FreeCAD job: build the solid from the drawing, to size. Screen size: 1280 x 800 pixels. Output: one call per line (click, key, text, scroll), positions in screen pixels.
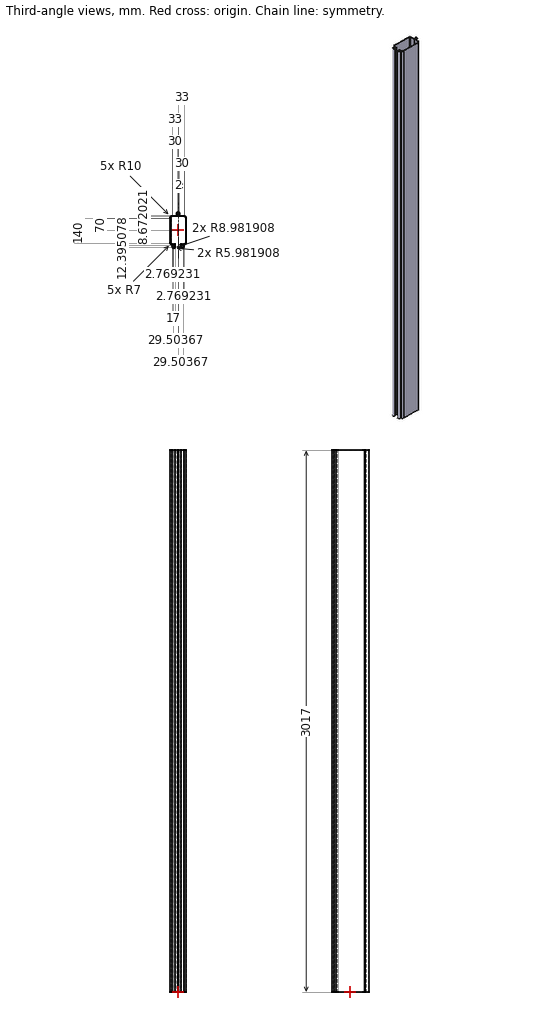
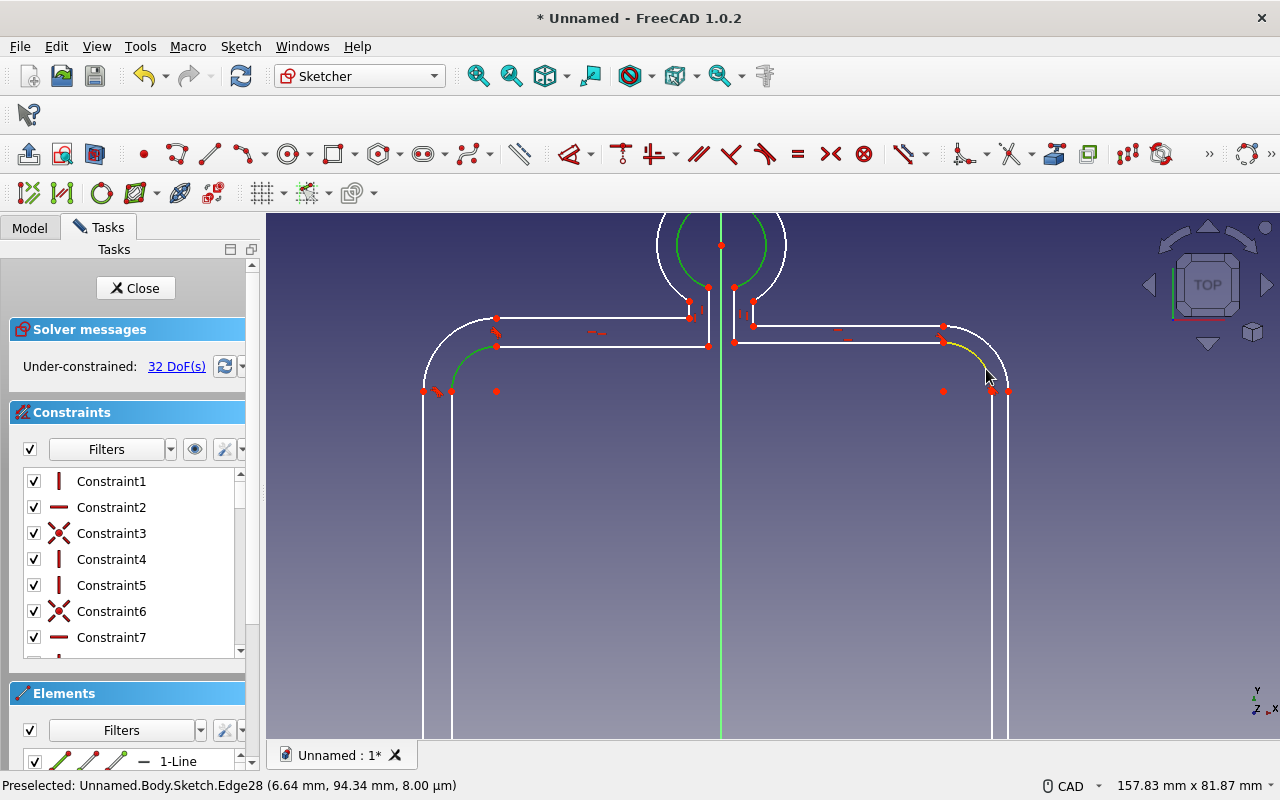
click(986, 369)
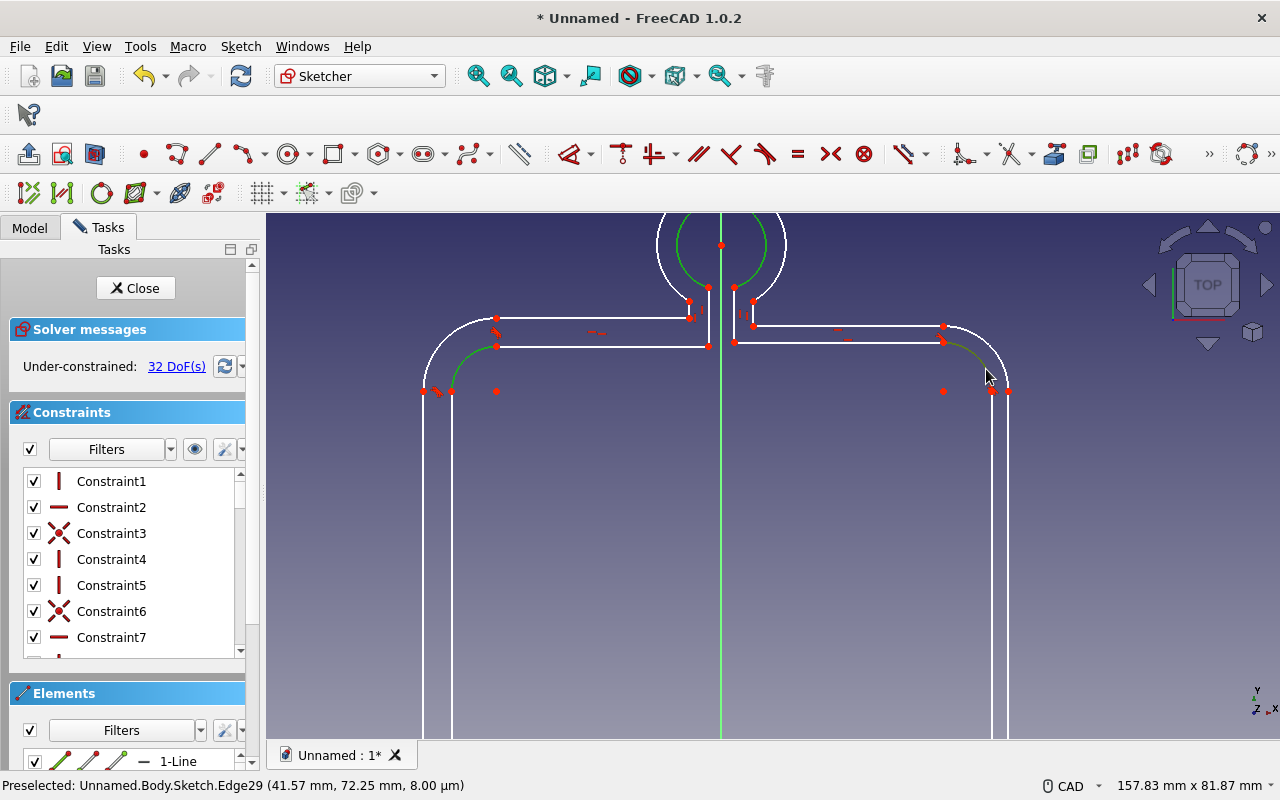
scroll(699, 359, down, 7)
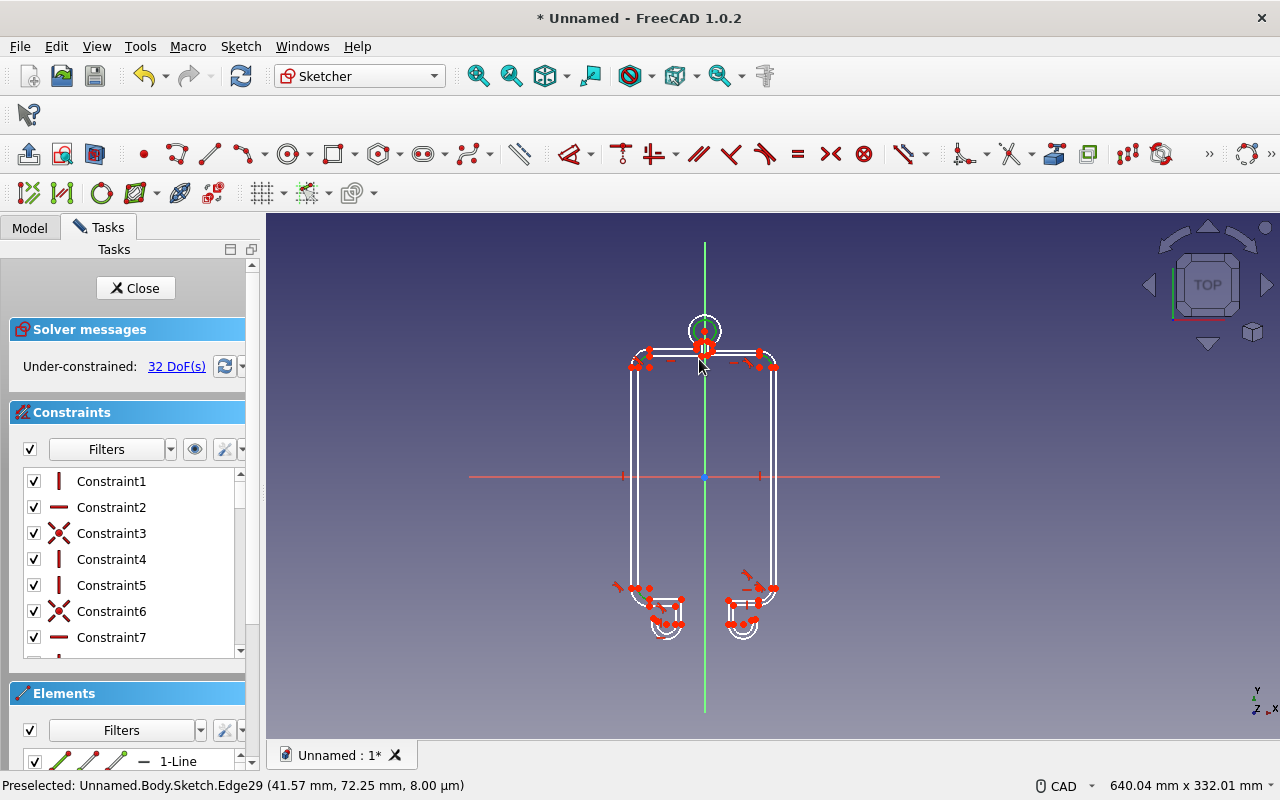
scroll(765, 600, up, 7)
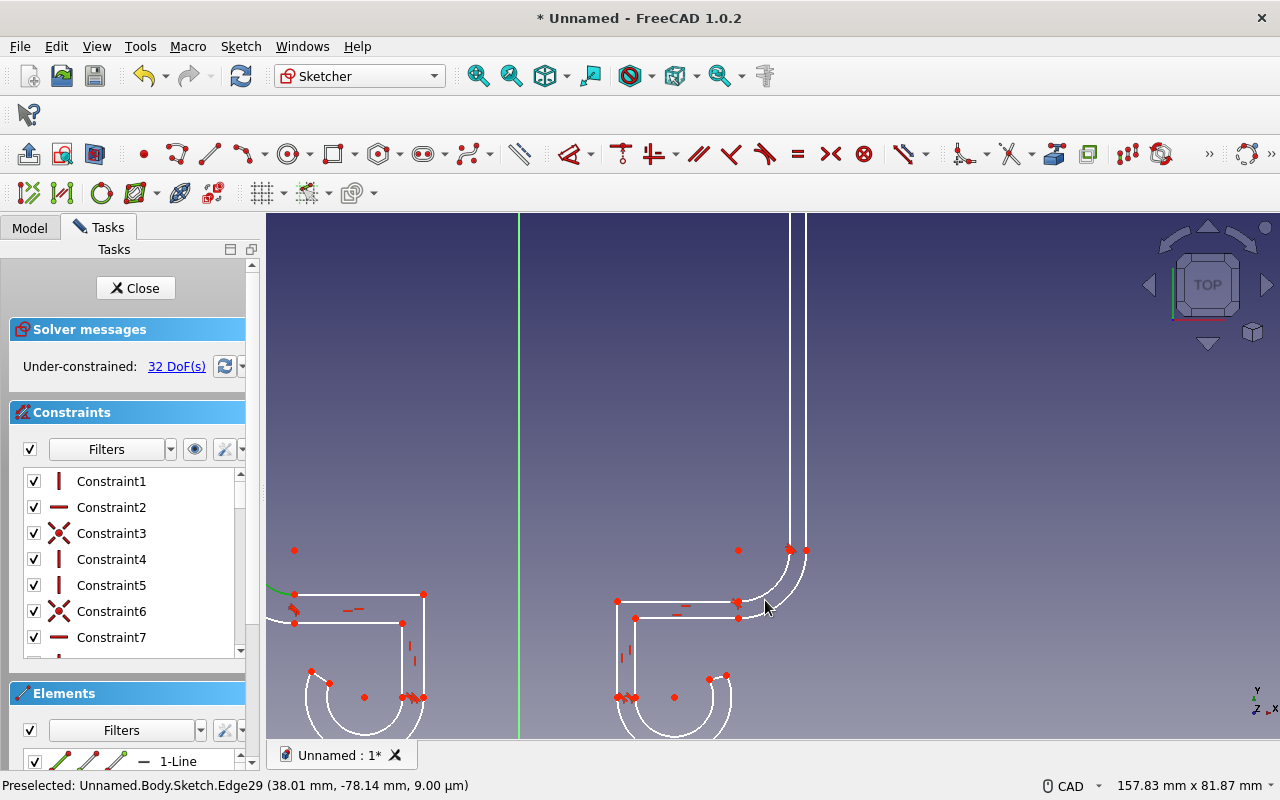
click(762, 596)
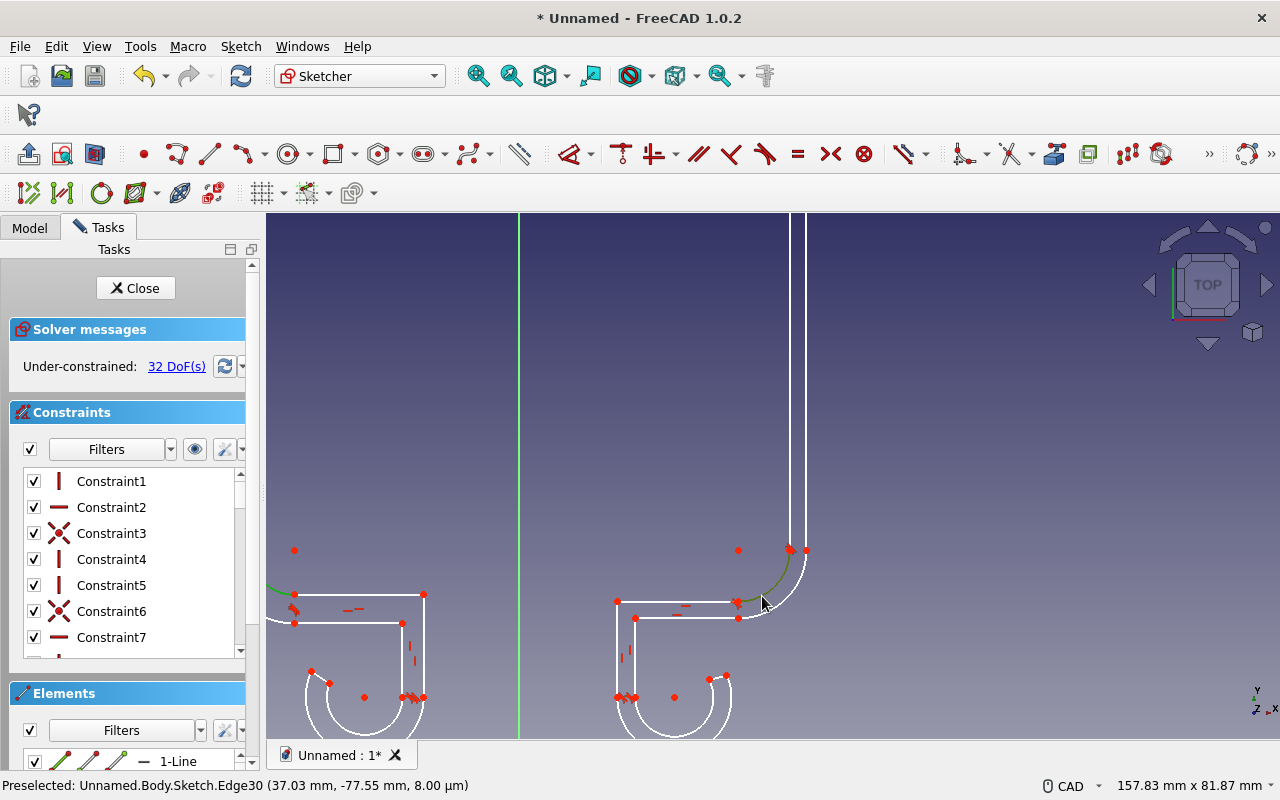
click(798, 154)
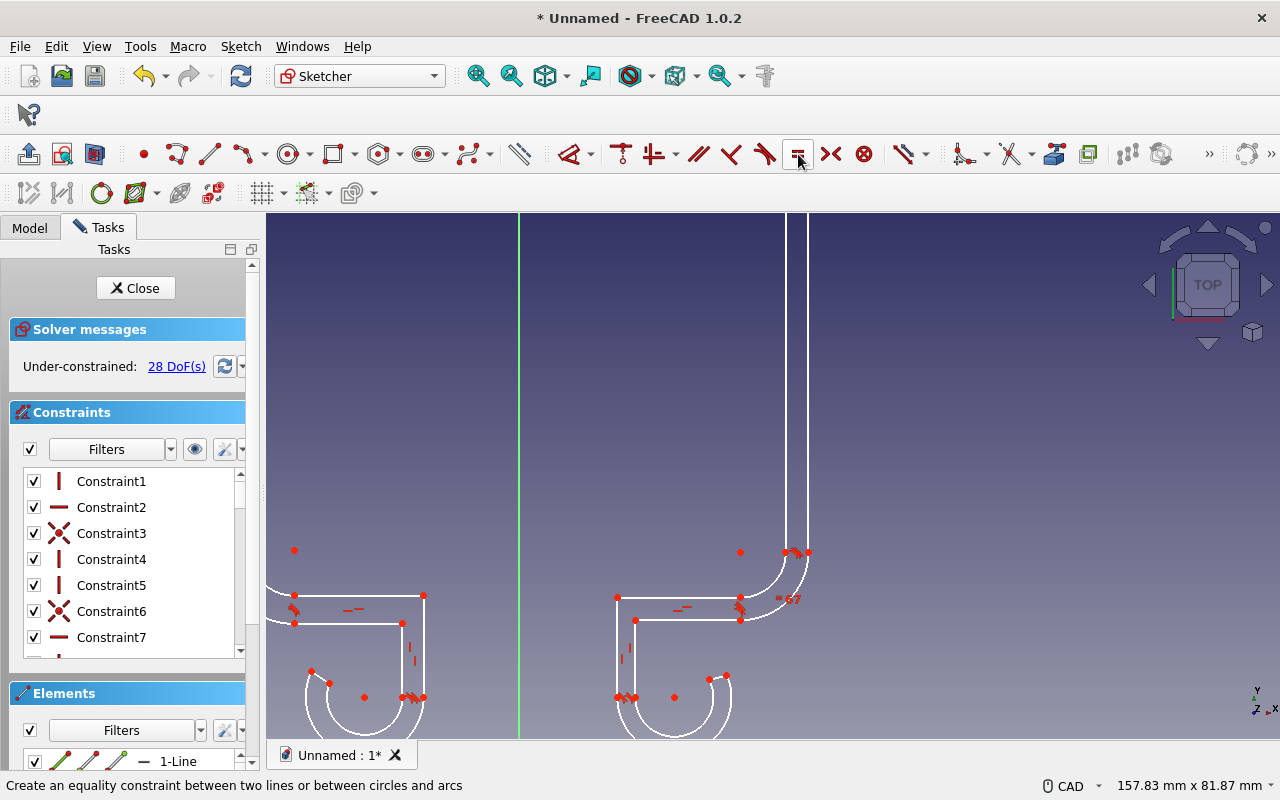
scroll(765, 600, down, 7)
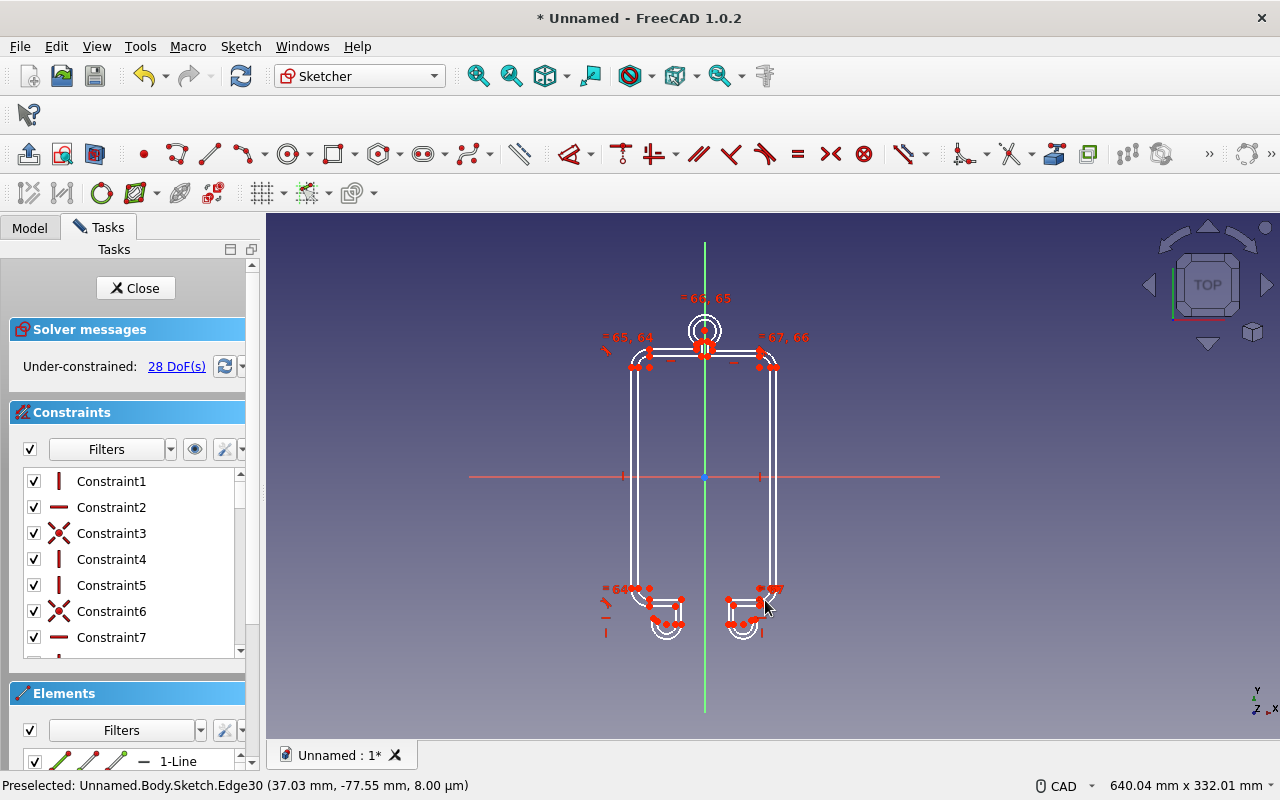
scroll(655, 633, up, 5)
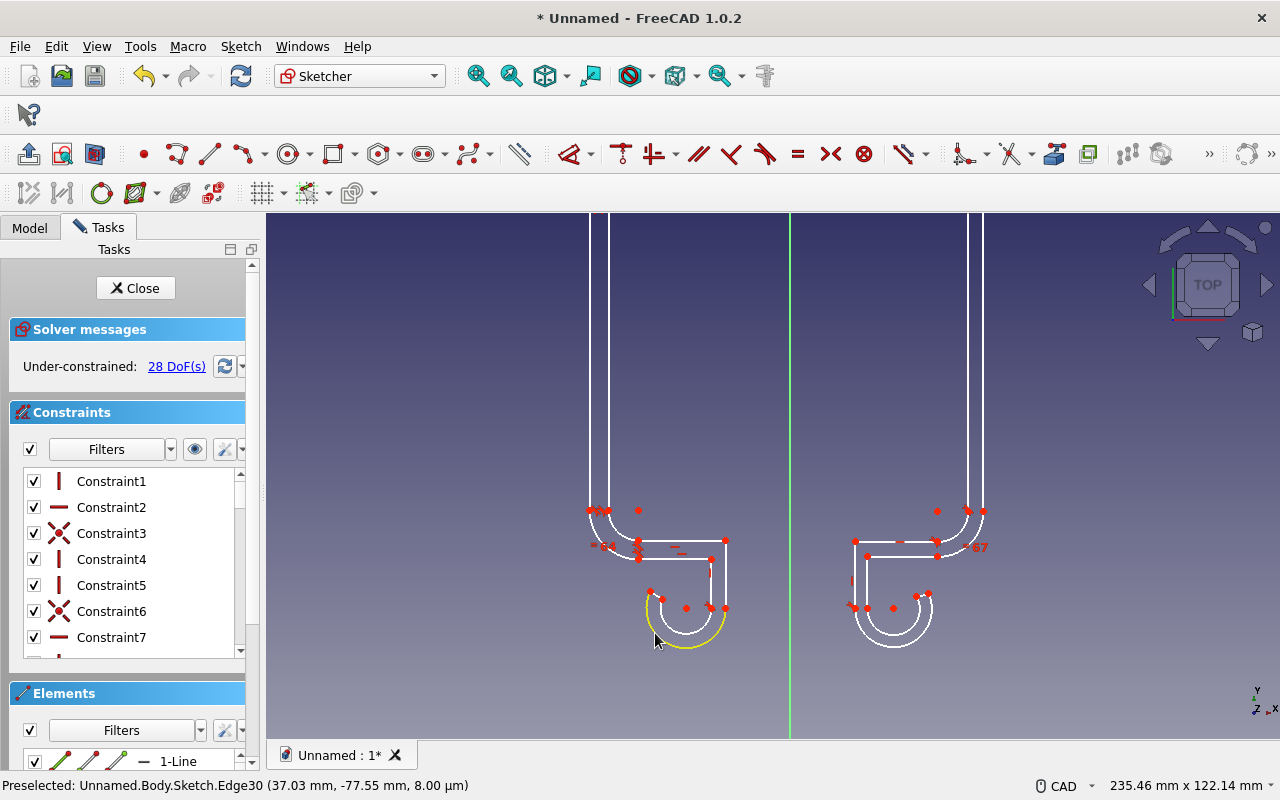
click(654, 632)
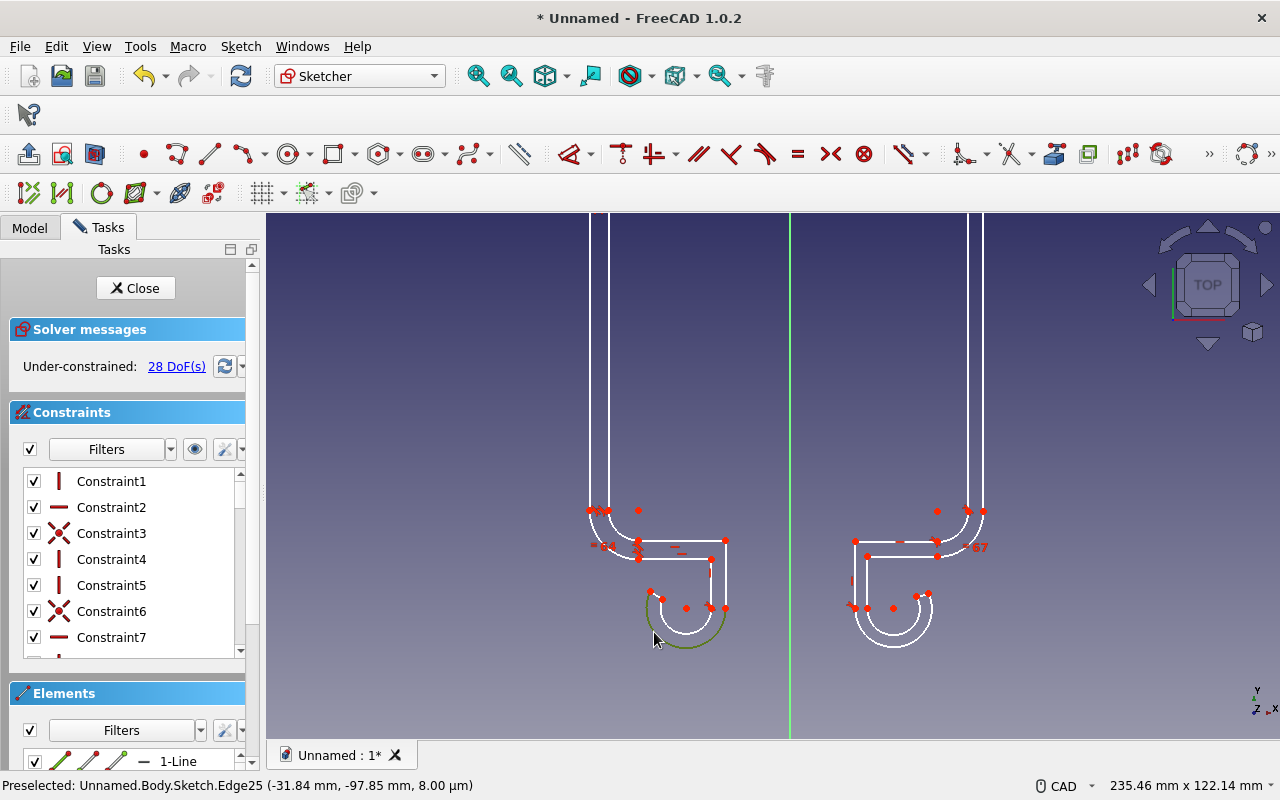
click(875, 642)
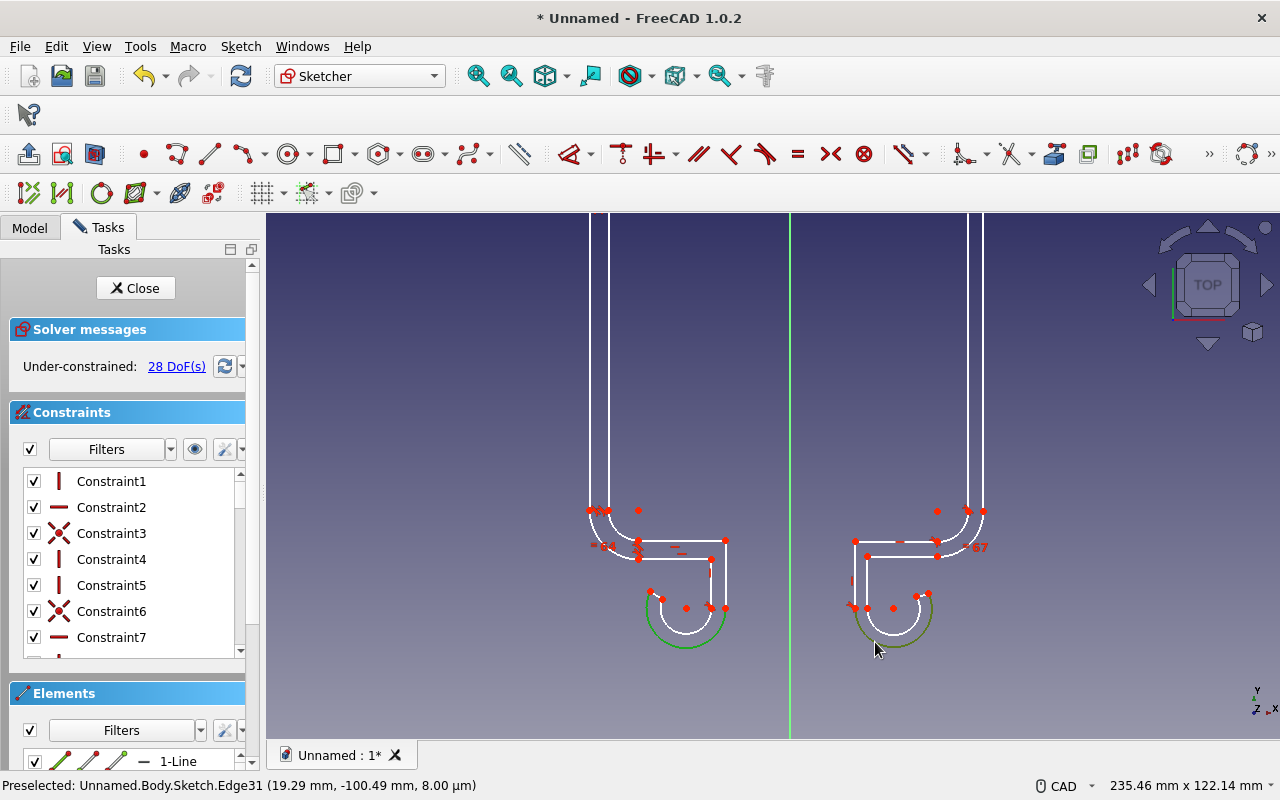
click(798, 154)